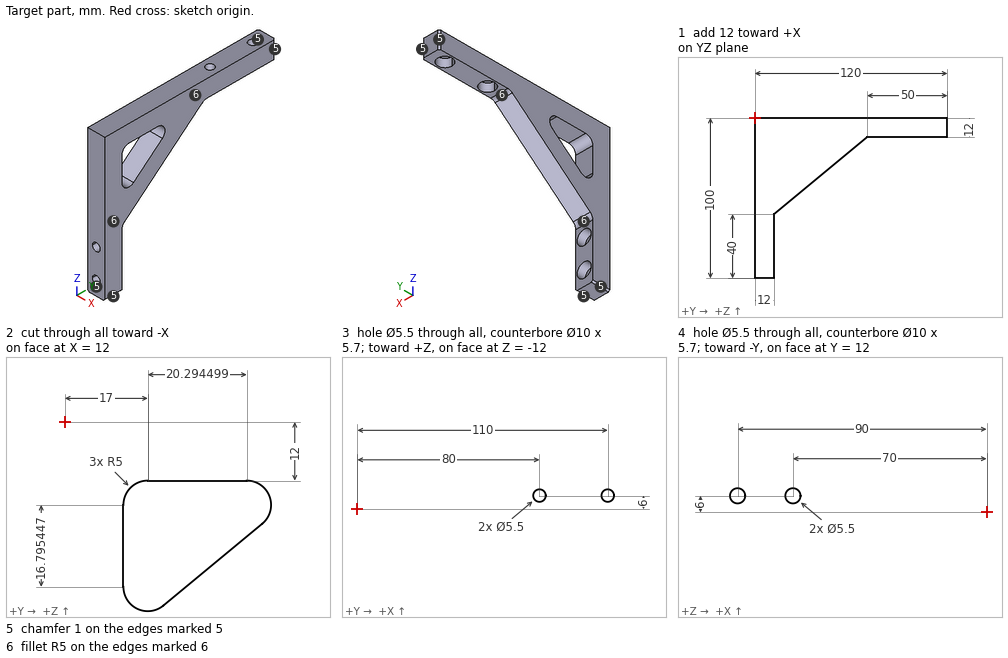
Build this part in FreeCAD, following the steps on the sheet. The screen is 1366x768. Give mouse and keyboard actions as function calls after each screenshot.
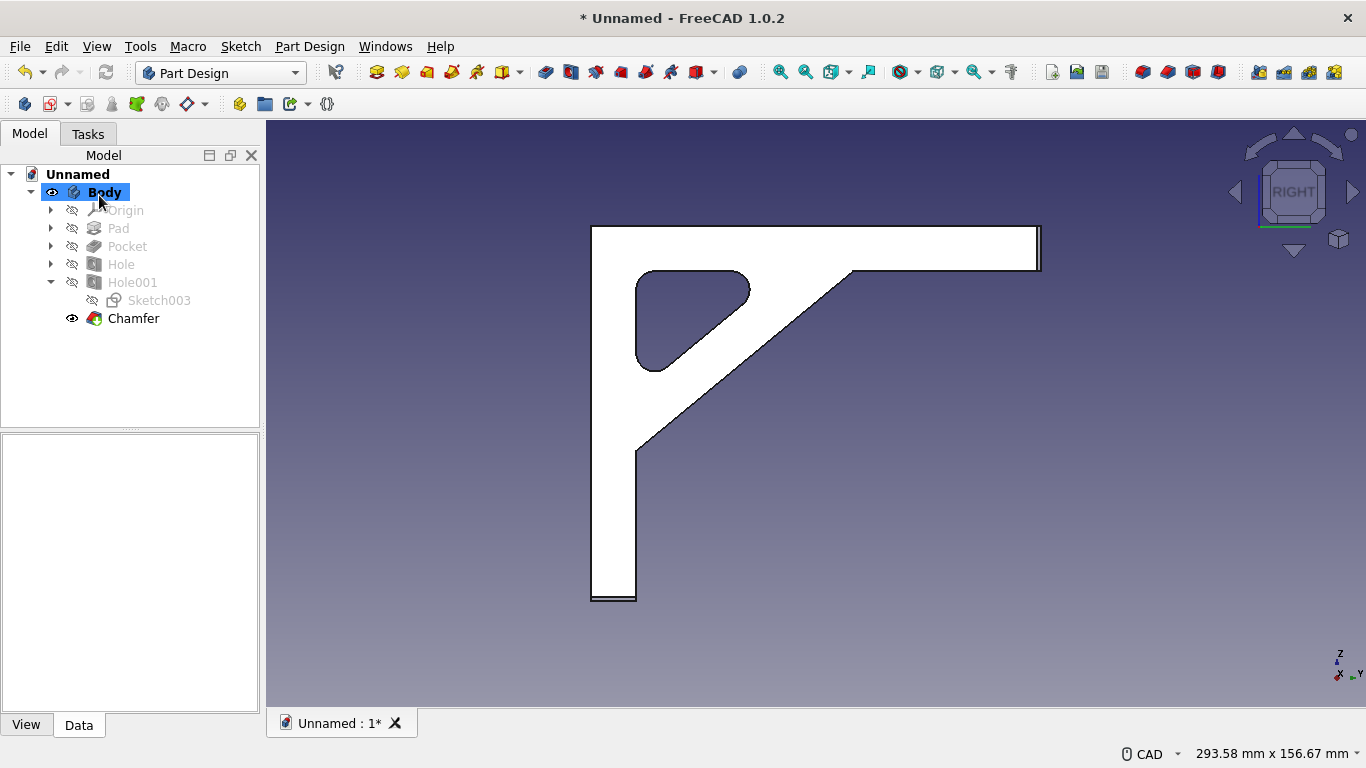
key(5)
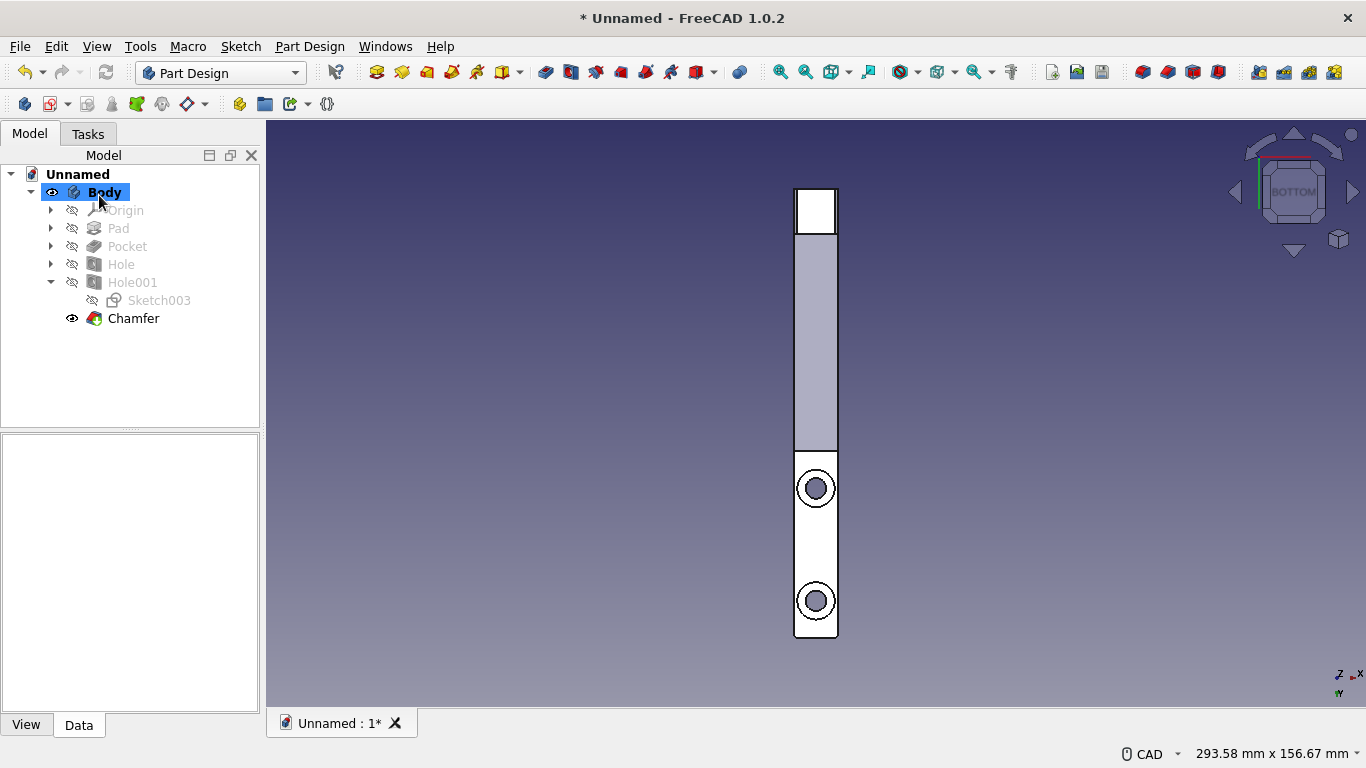
key(4)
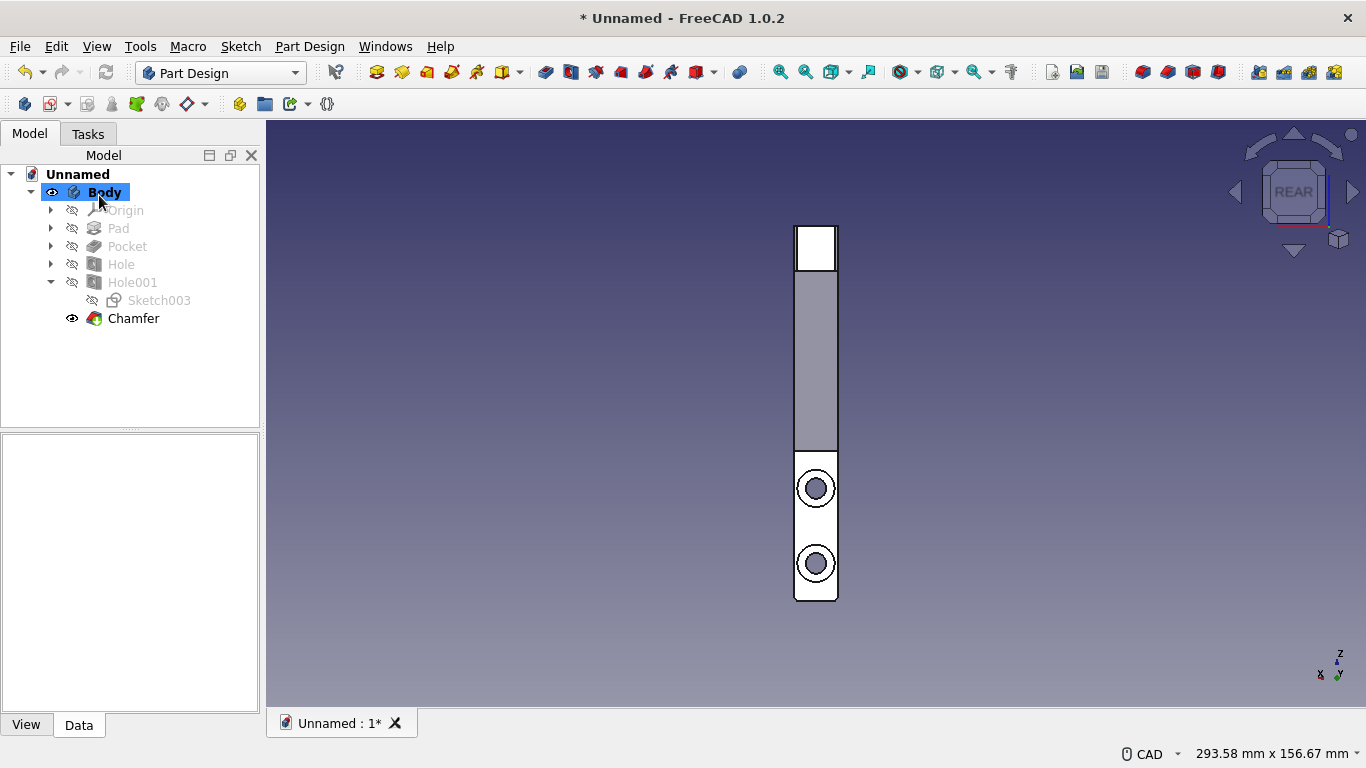
key(6)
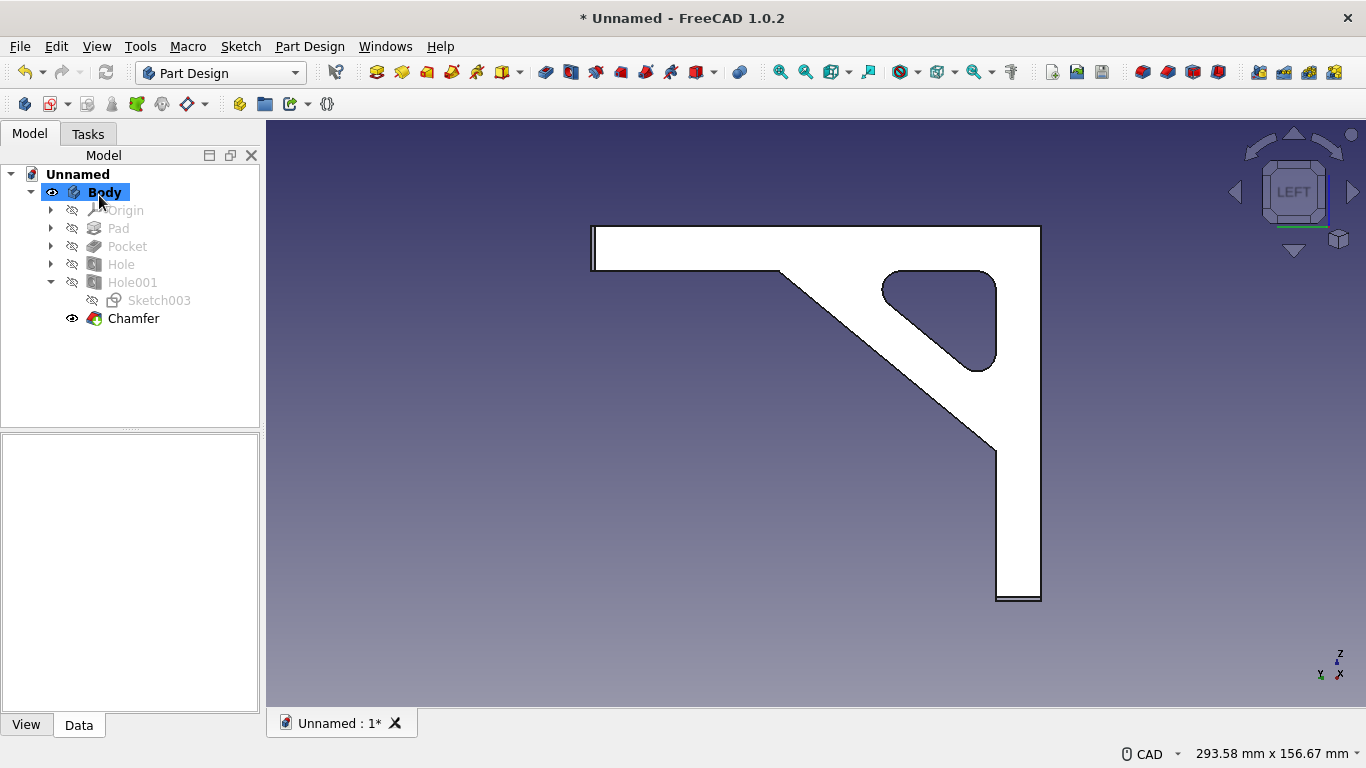
key(v)
key(3)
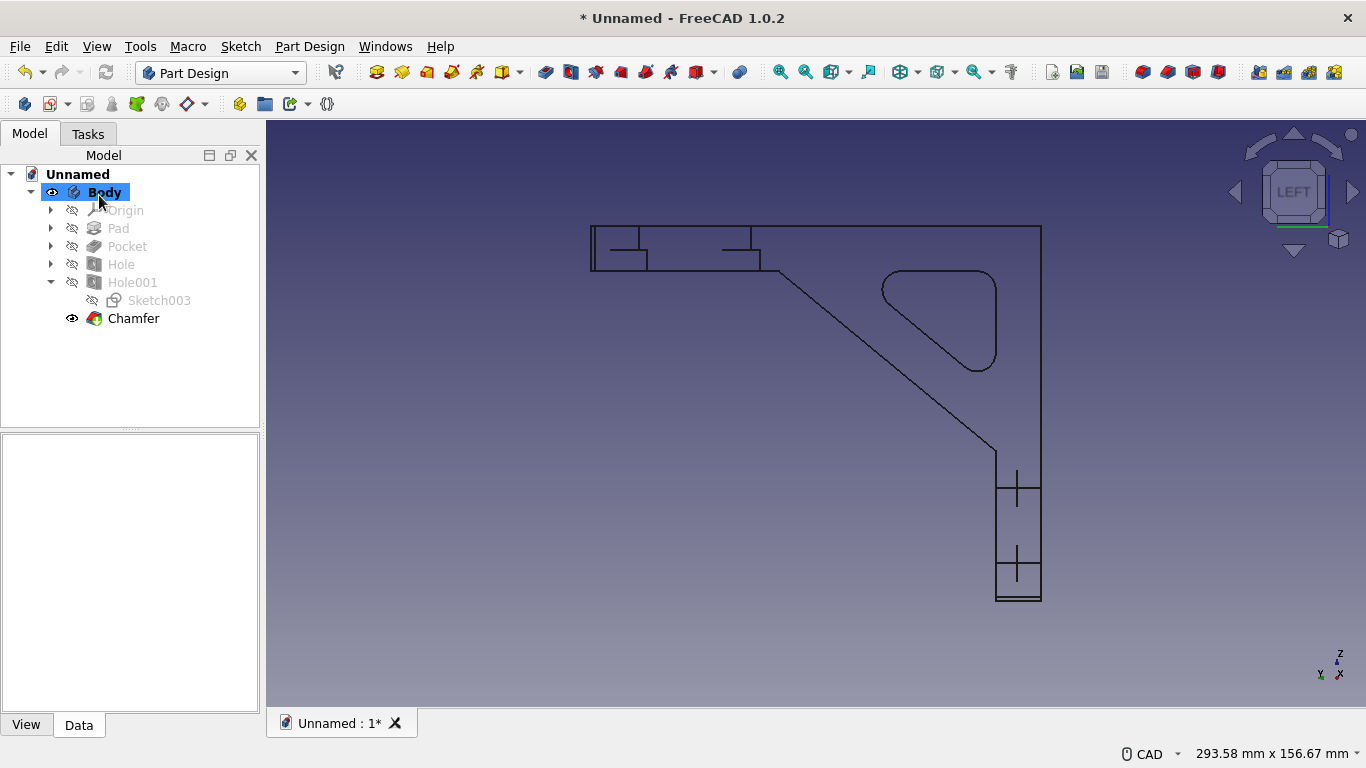
key(0)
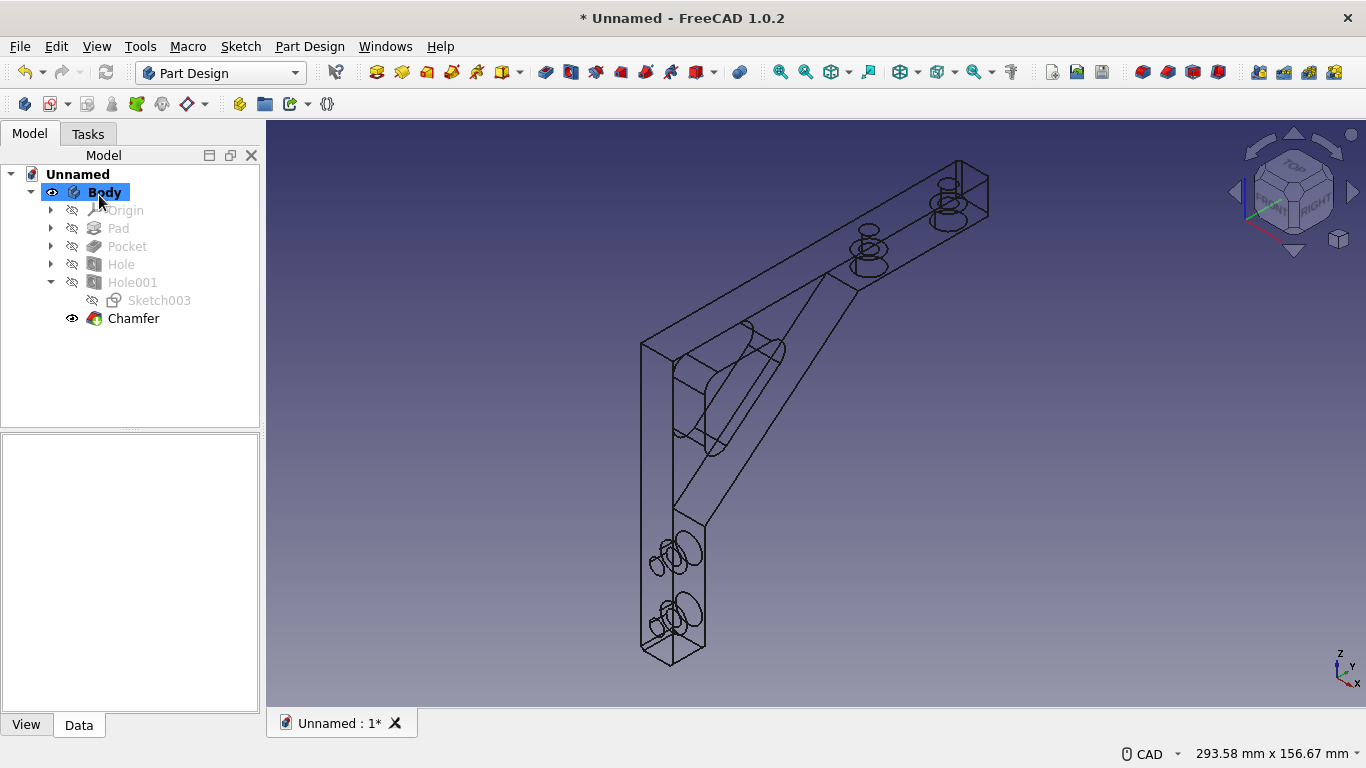
click(842, 281)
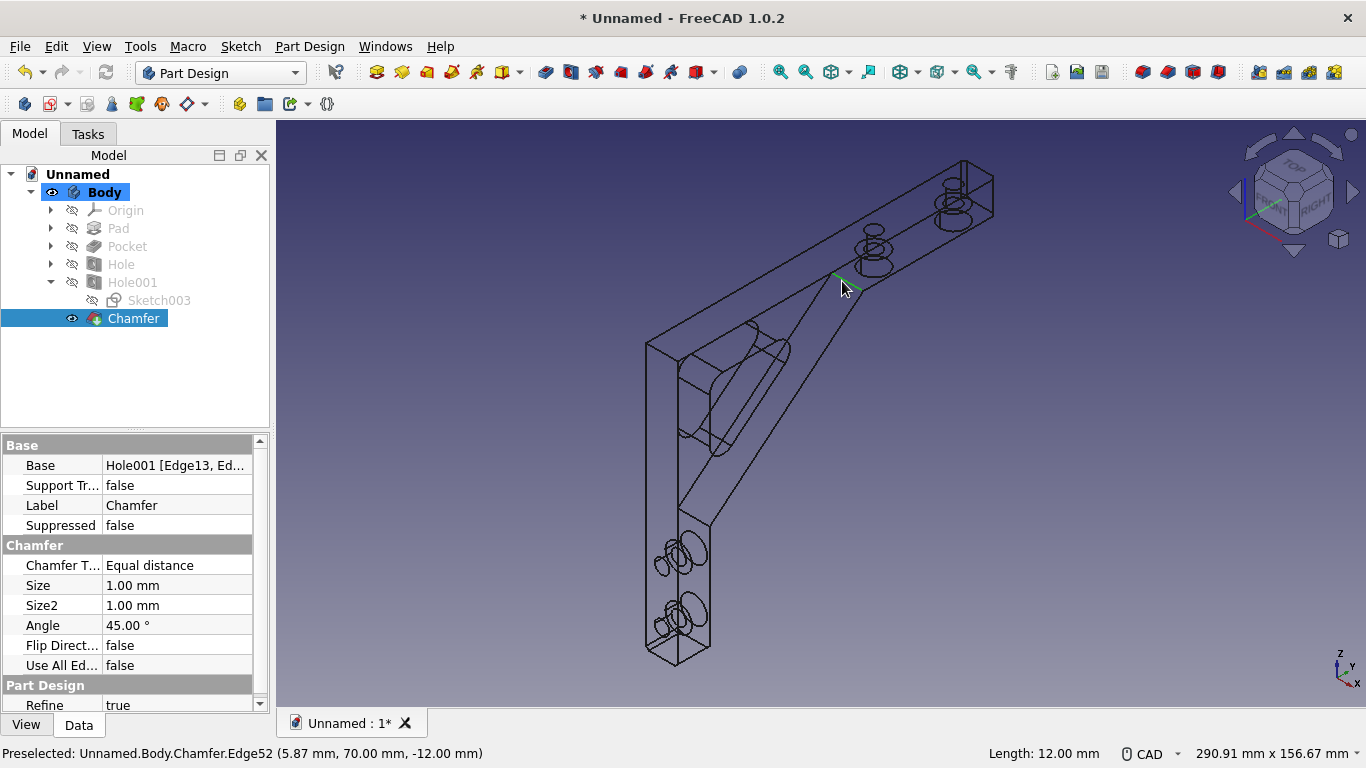
click(694, 517, ctrl)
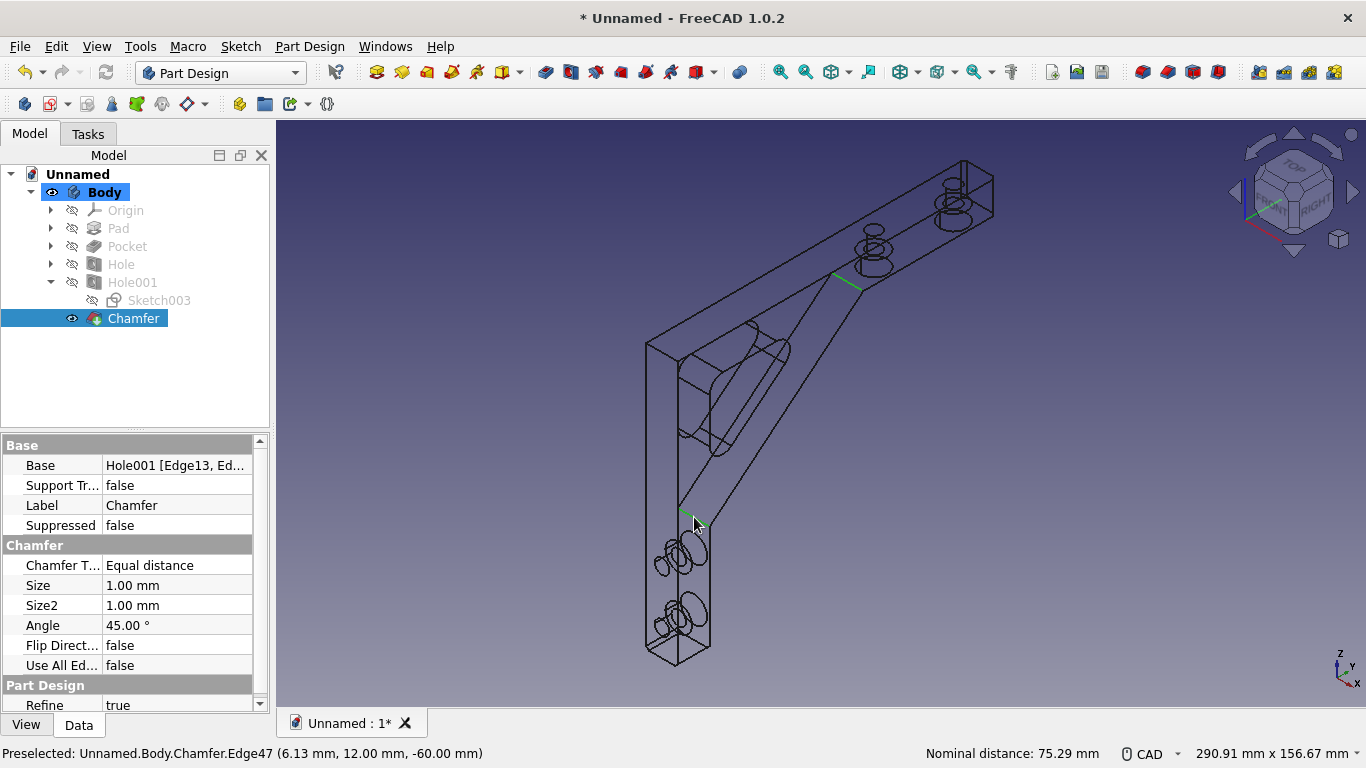
key(v)
key(1)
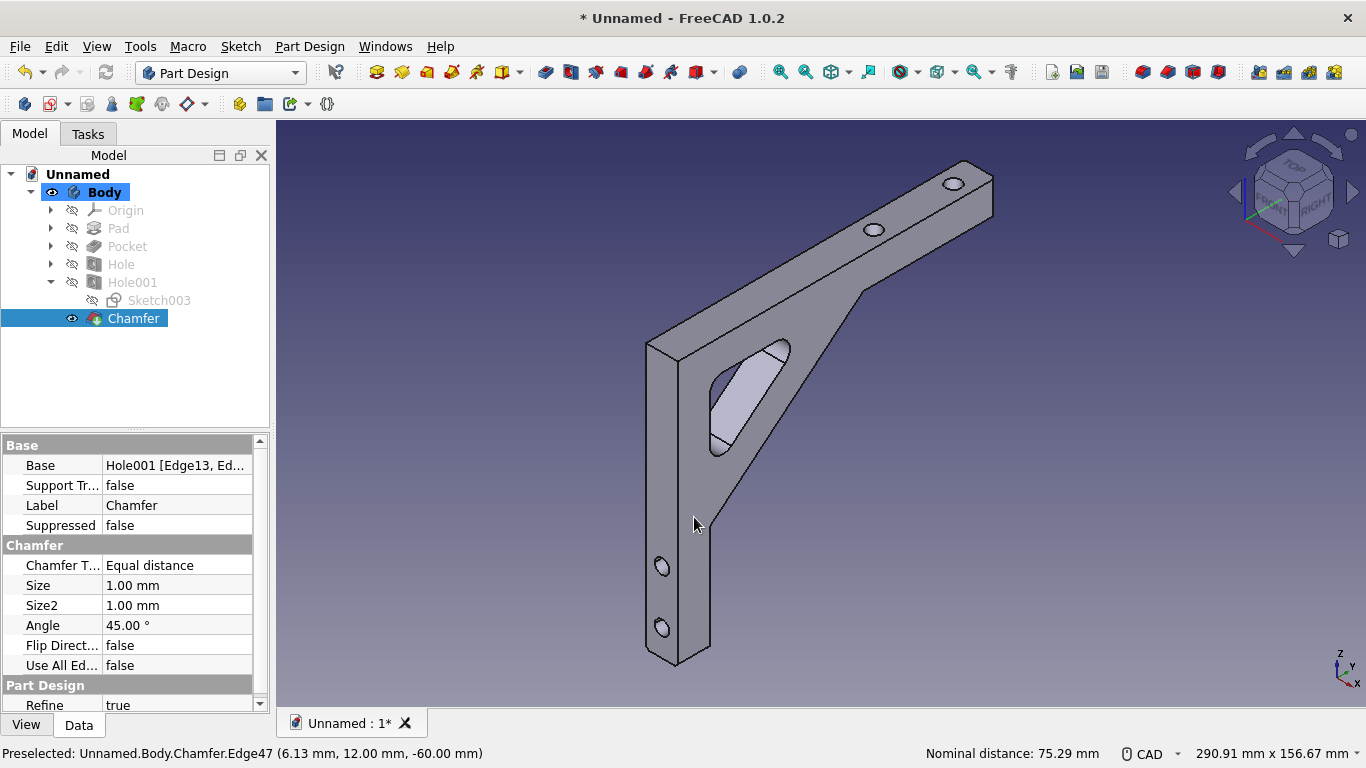
click(1143, 72)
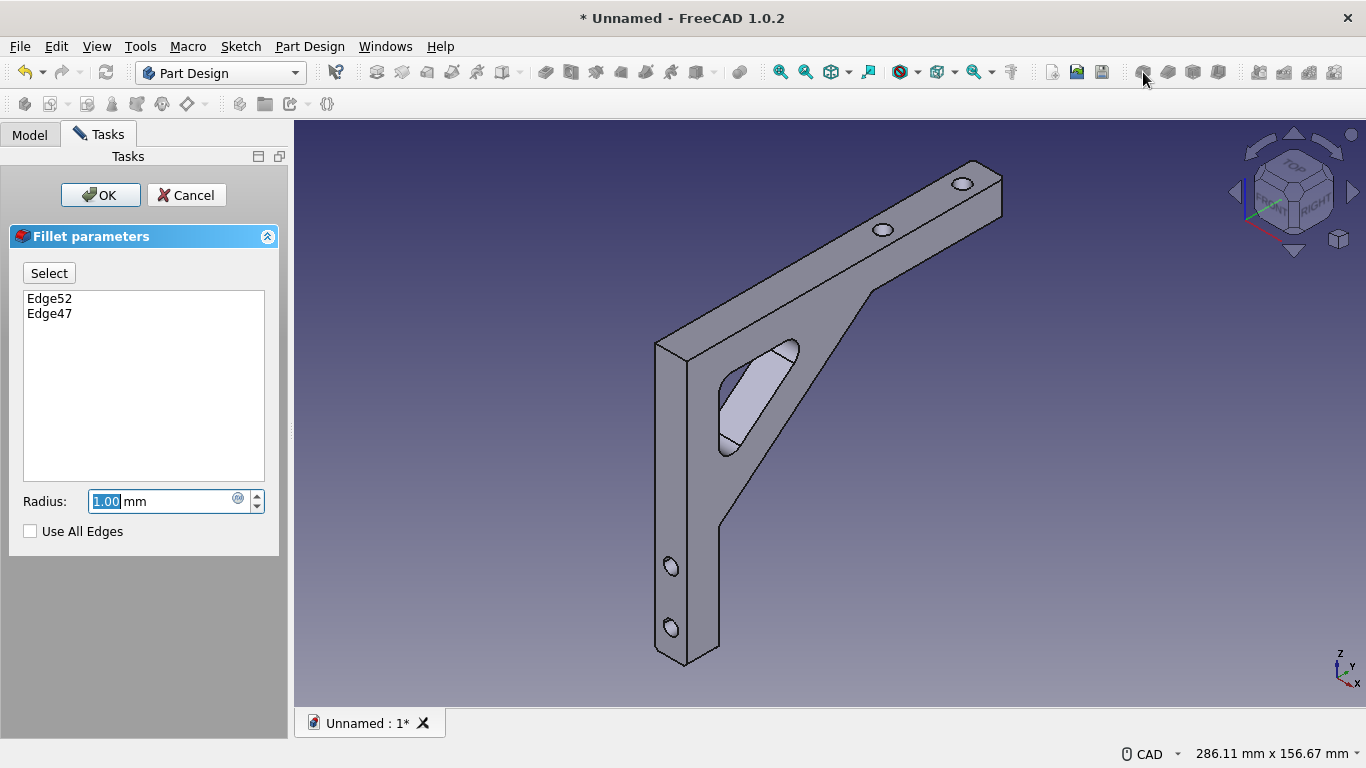
text(5)
key(Tab)